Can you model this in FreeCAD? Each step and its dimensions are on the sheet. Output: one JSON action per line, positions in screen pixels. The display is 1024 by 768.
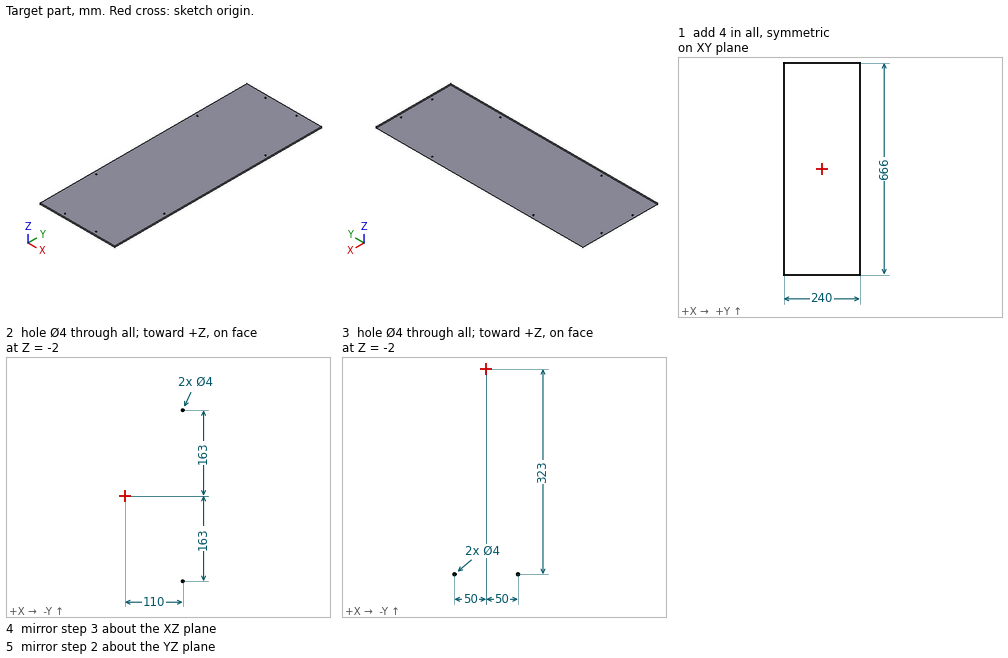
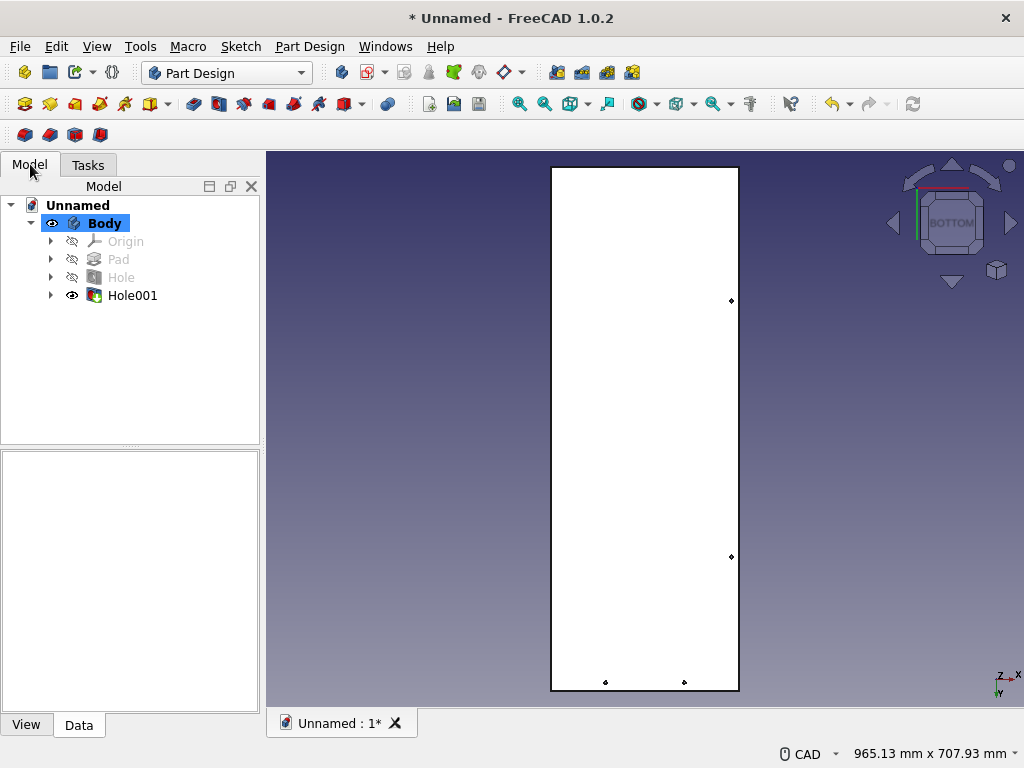
{"action": "left_click", "coordinate": [117, 295]}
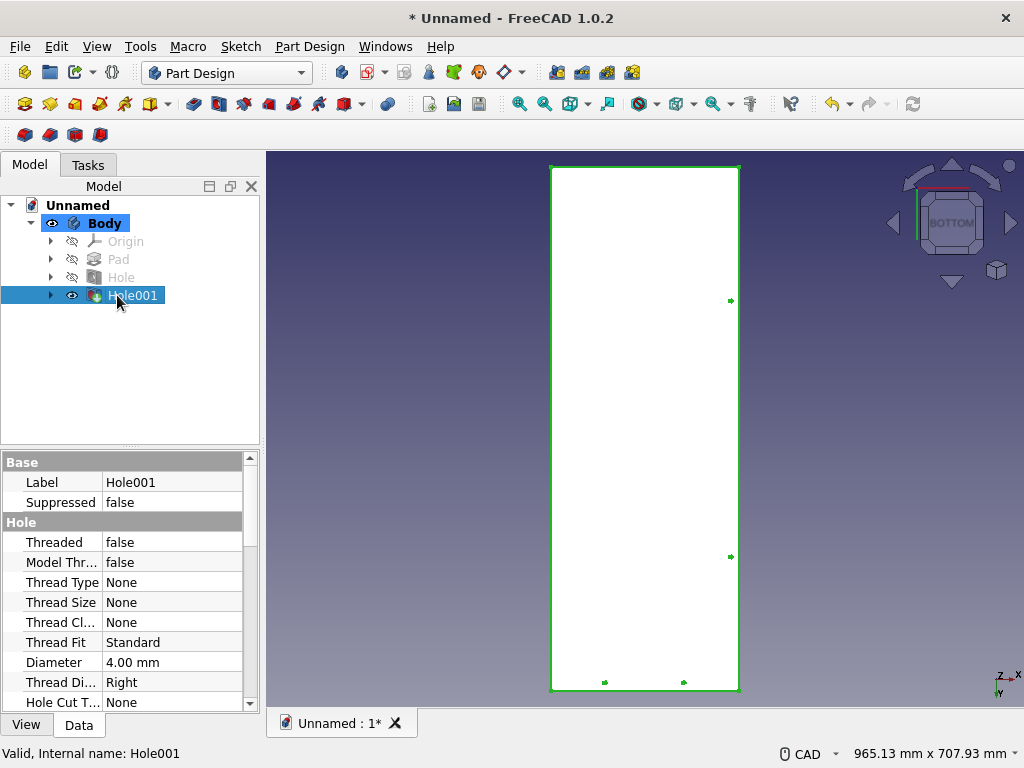
{"action": "left_click", "coordinate": [557, 72]}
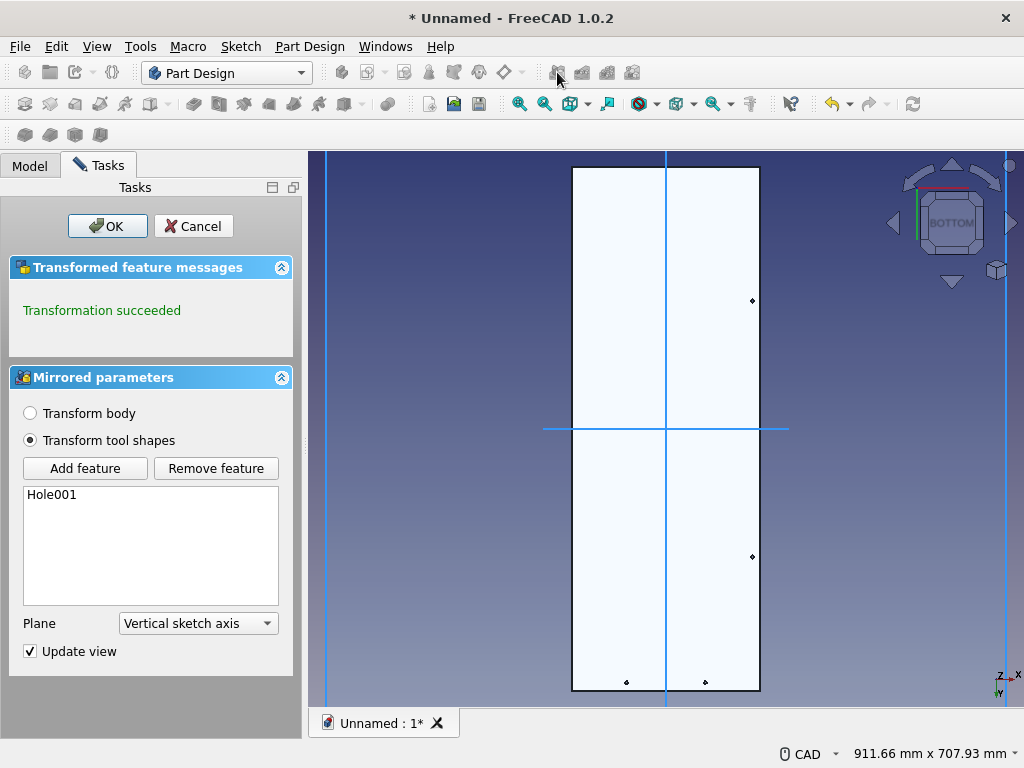
{"action": "left_click", "coordinate": [199, 624]}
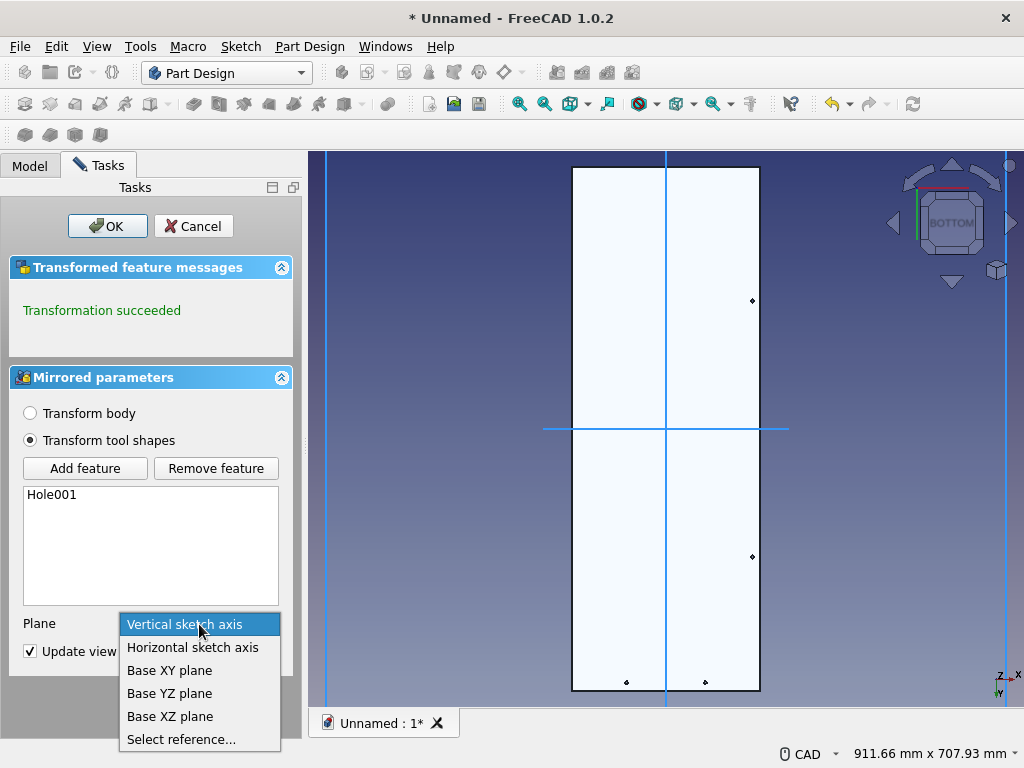
{"action": "left_click", "coordinate": [198, 716]}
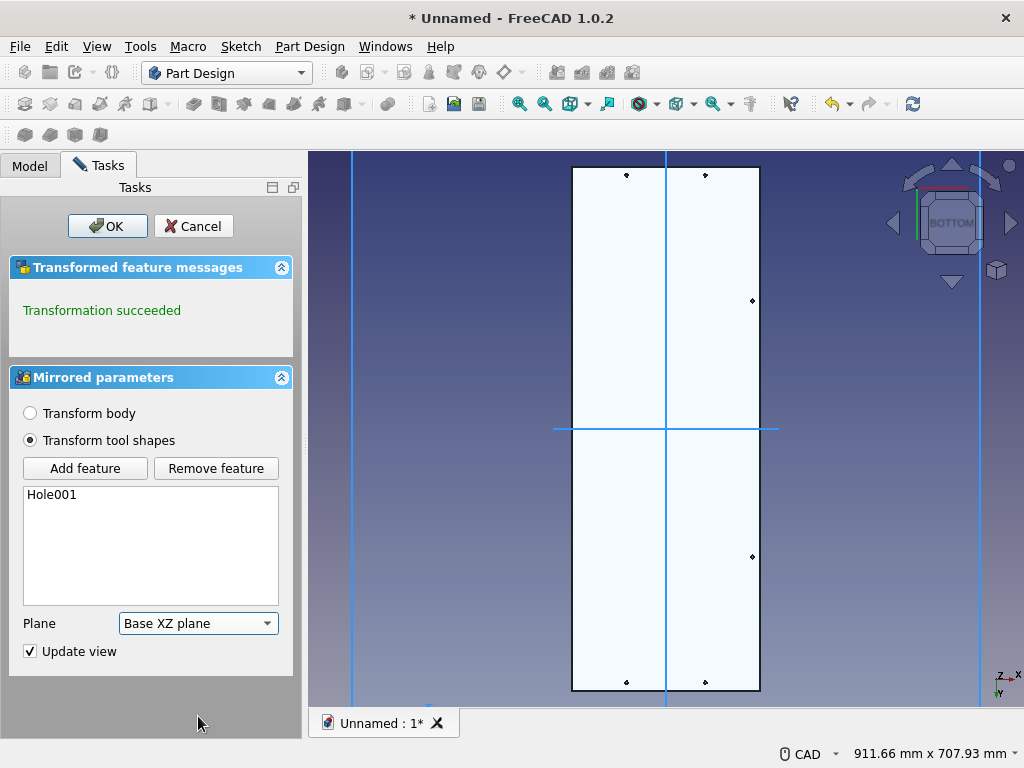
{"action": "left_click", "coordinate": [108, 226]}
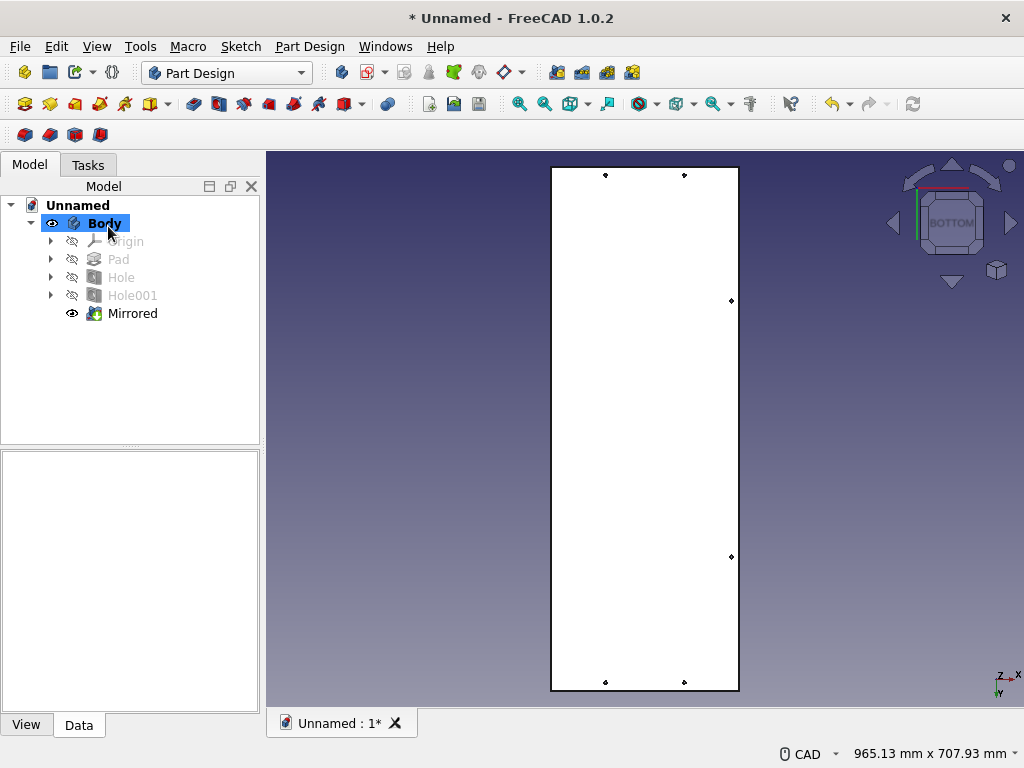
{"action": "left_click", "coordinate": [117, 277]}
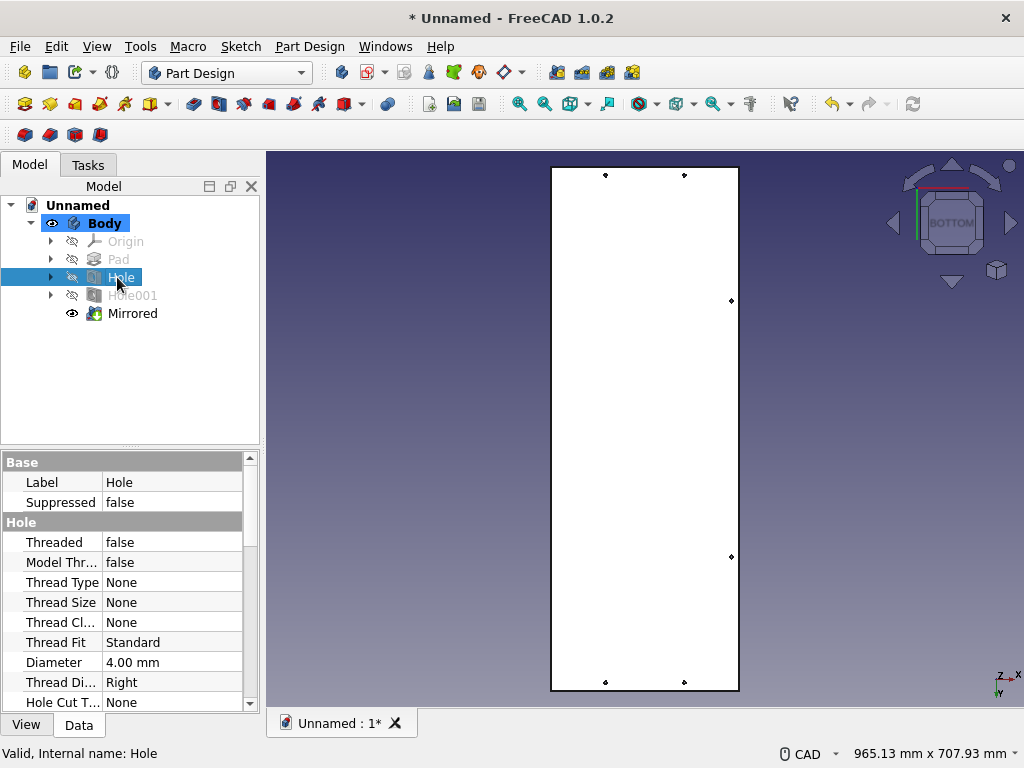
{"action": "left_click", "coordinate": [557, 72]}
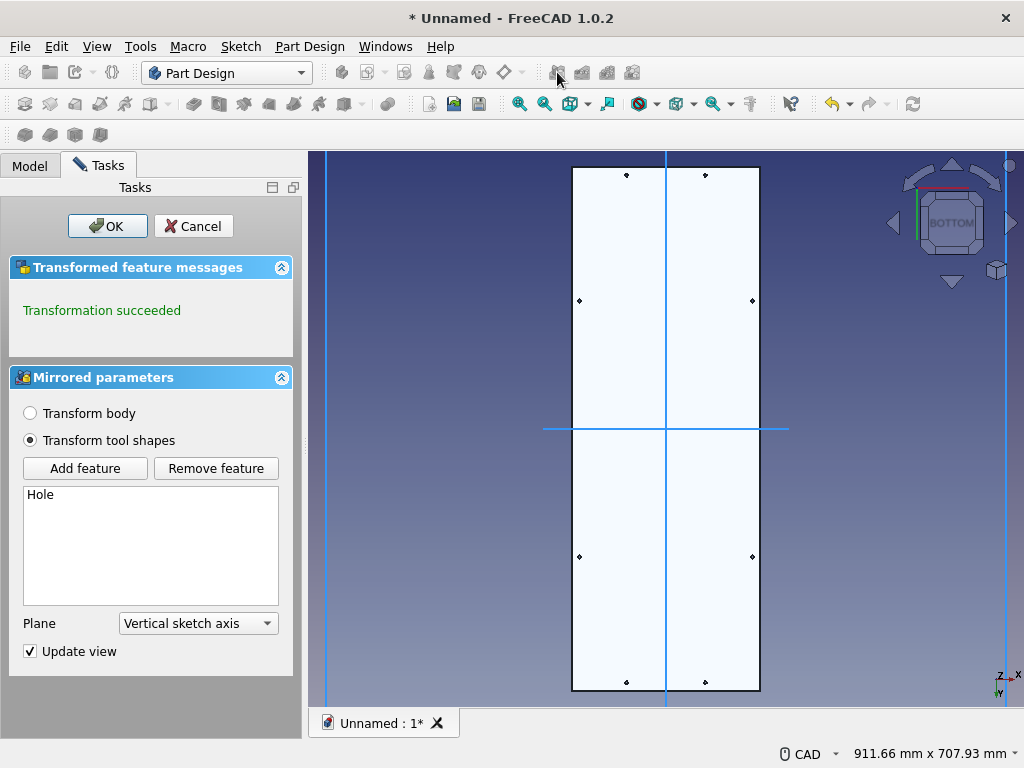
{"action": "left_click", "coordinate": [199, 624]}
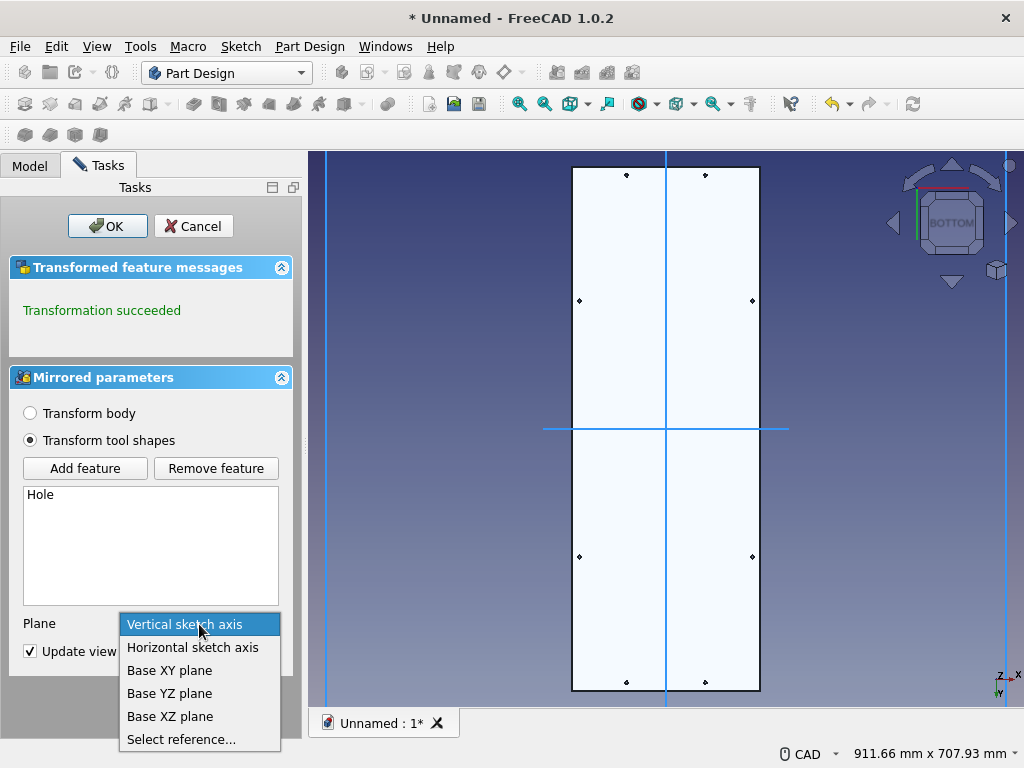
{"action": "left_click", "coordinate": [198, 694]}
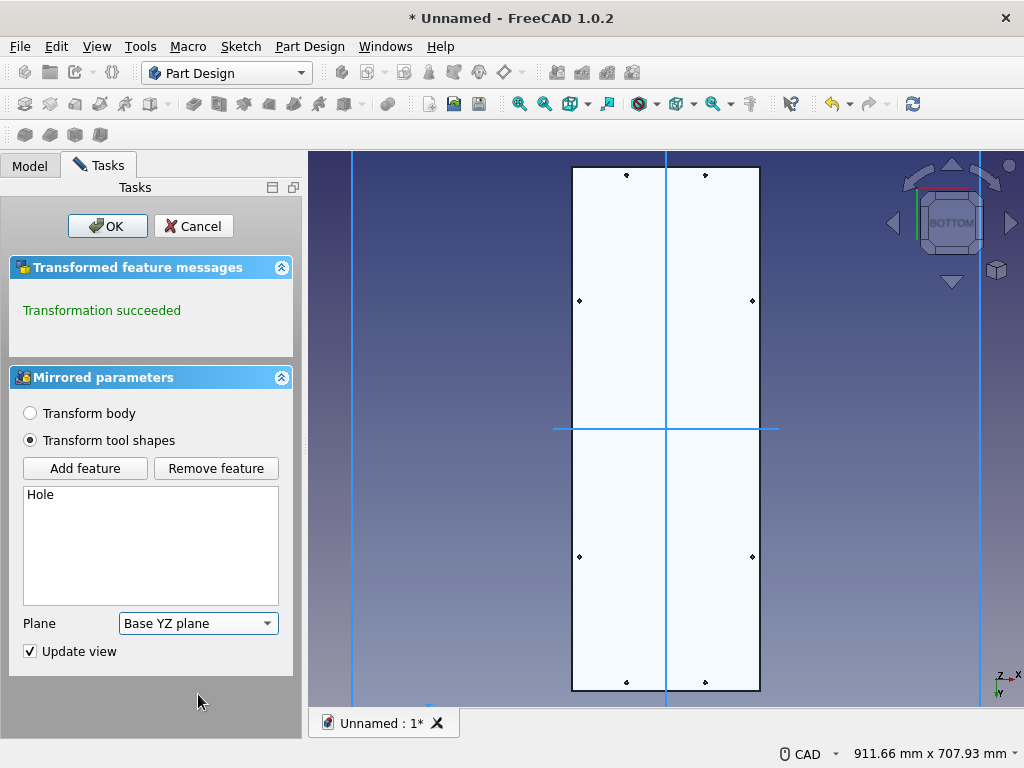
{"action": "left_click", "coordinate": [108, 226]}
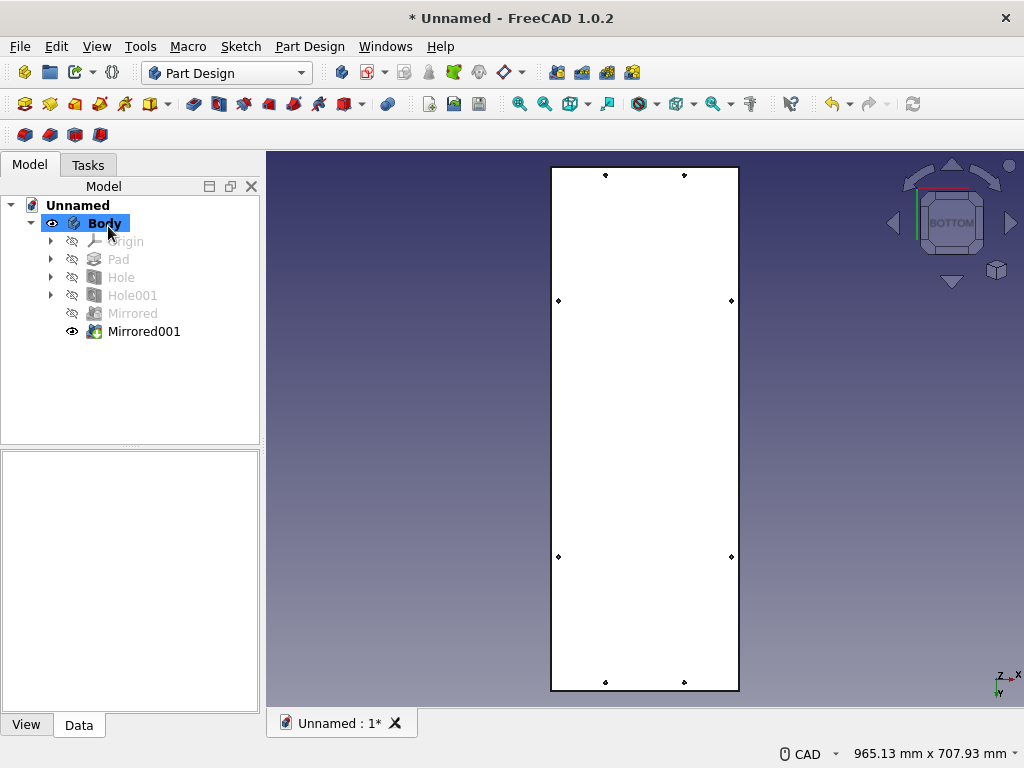
{"action": "key", "text": "0"}